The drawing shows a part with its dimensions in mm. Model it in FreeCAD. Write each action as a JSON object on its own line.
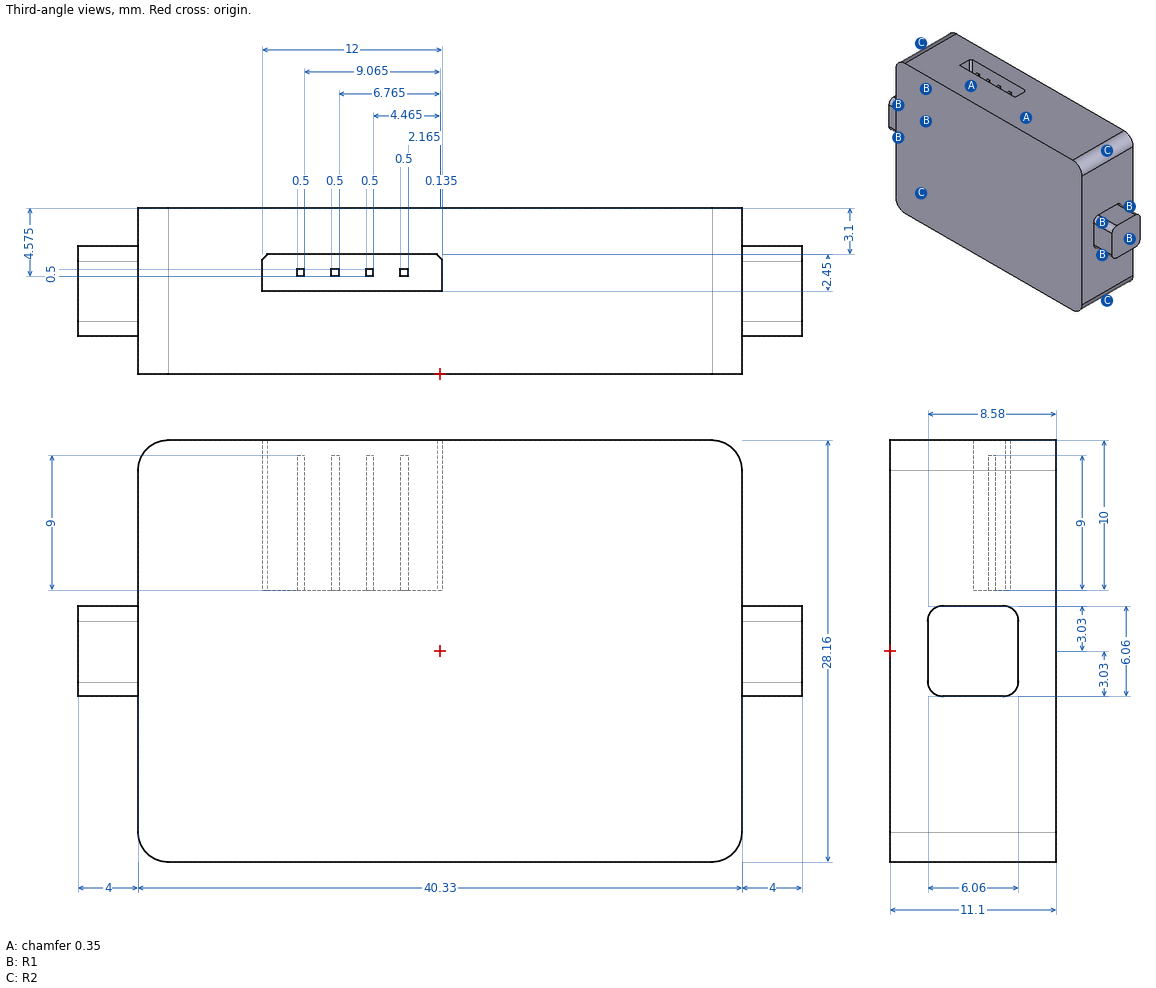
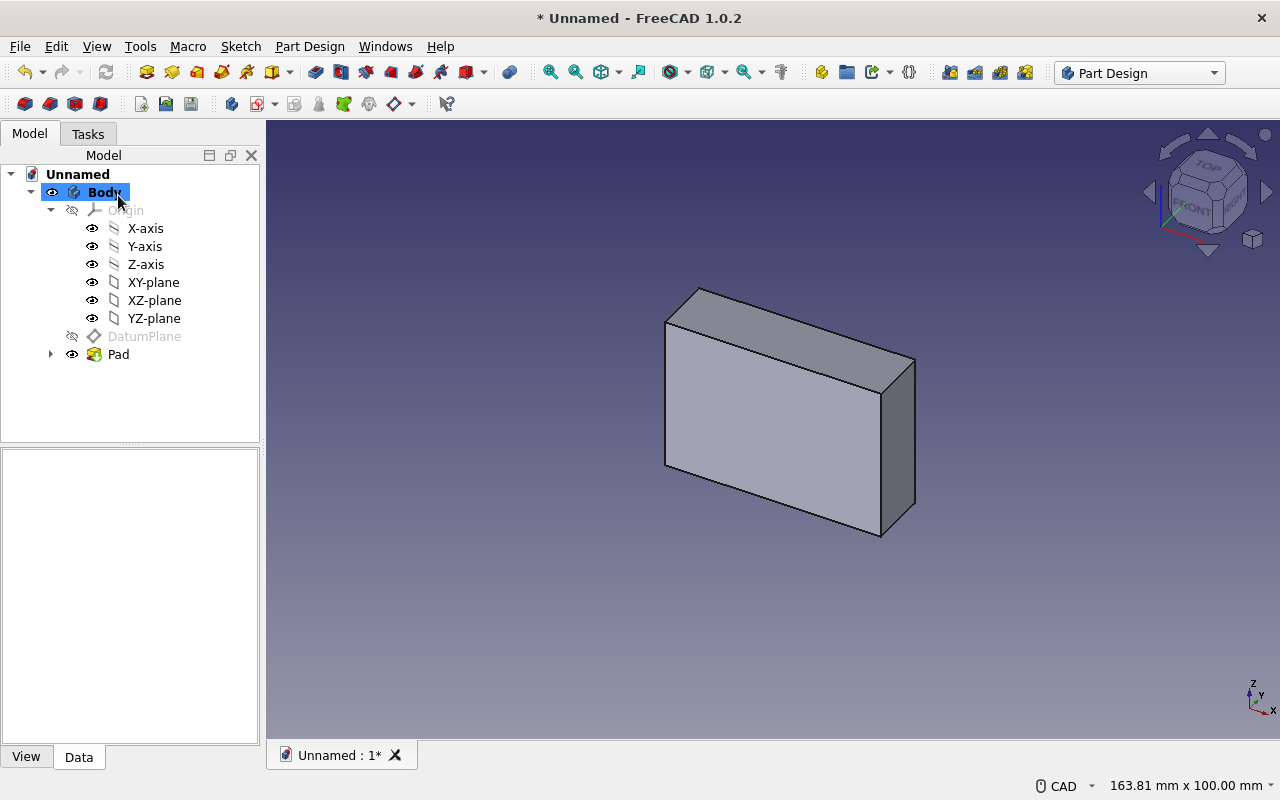
{"action": "key", "text": "v f"}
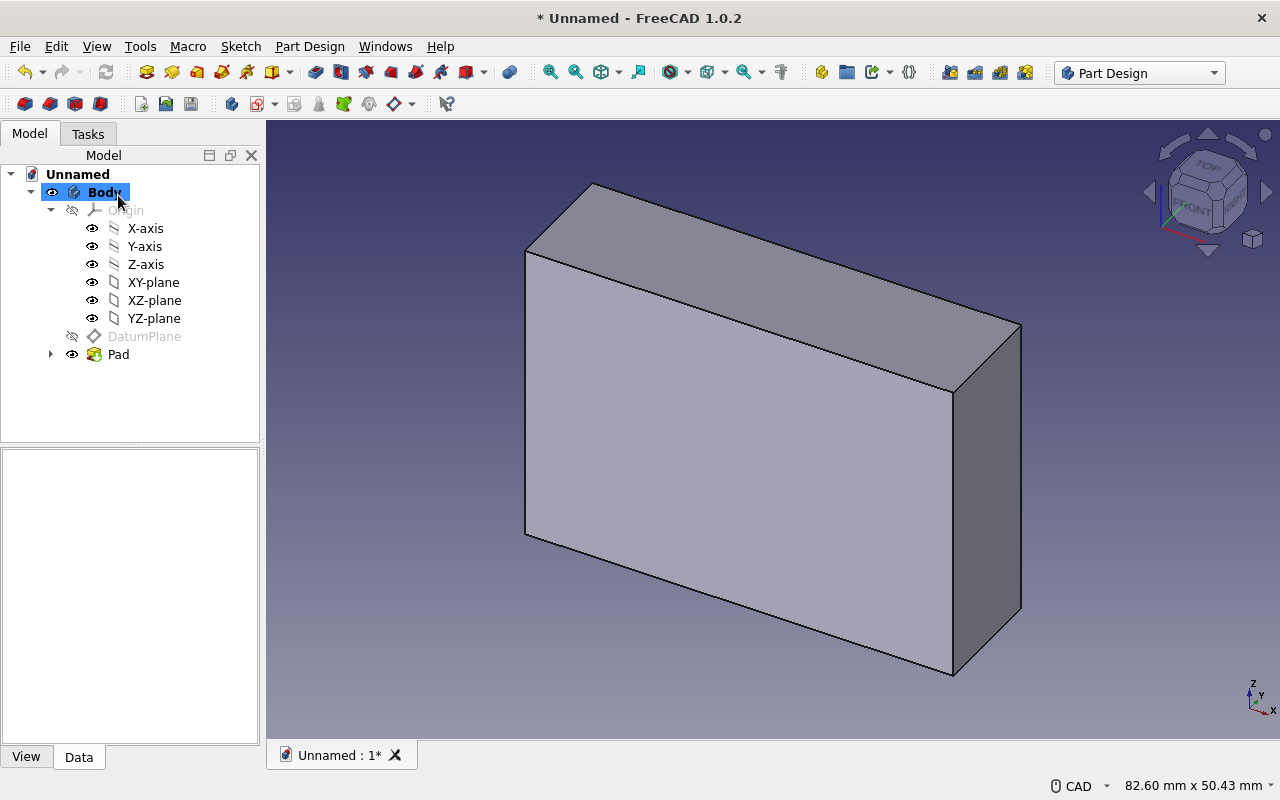
{"action": "left_click", "coordinate": [895, 327]}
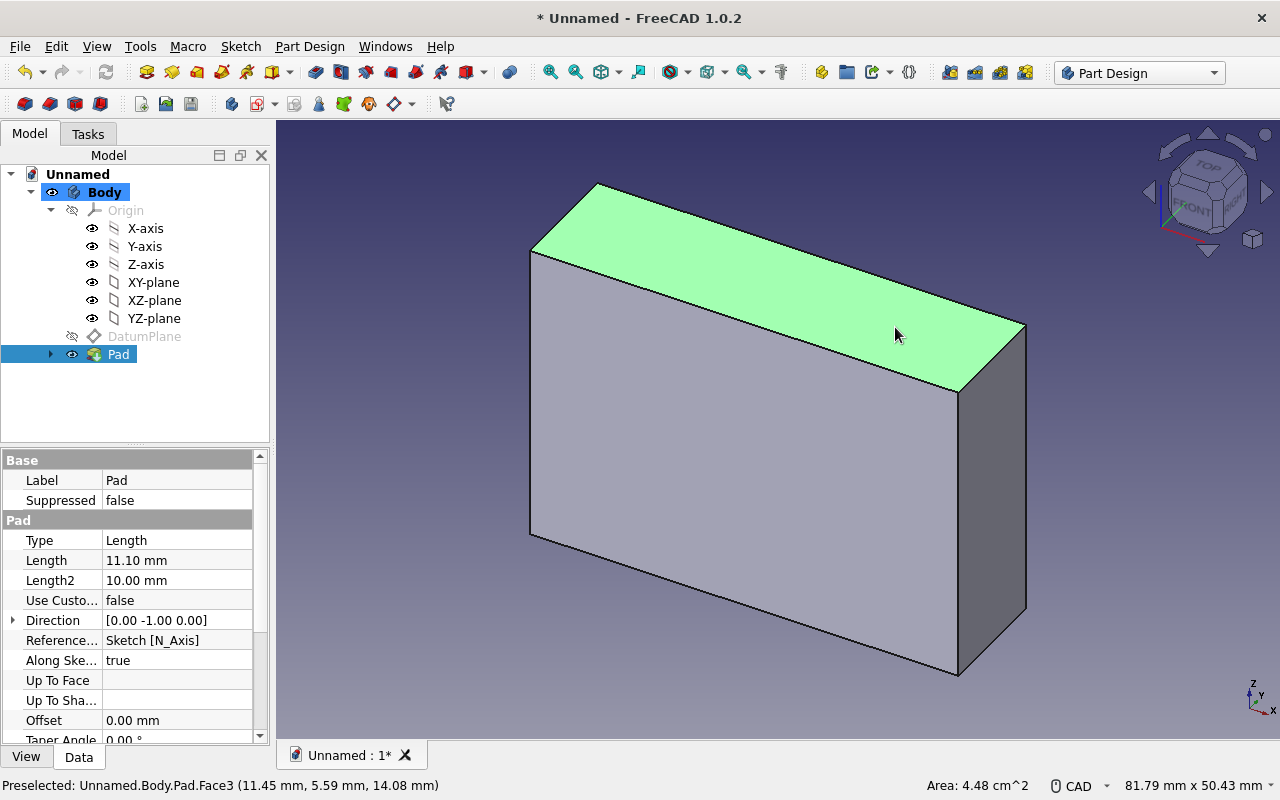
{"action": "left_click", "coordinate": [256, 104]}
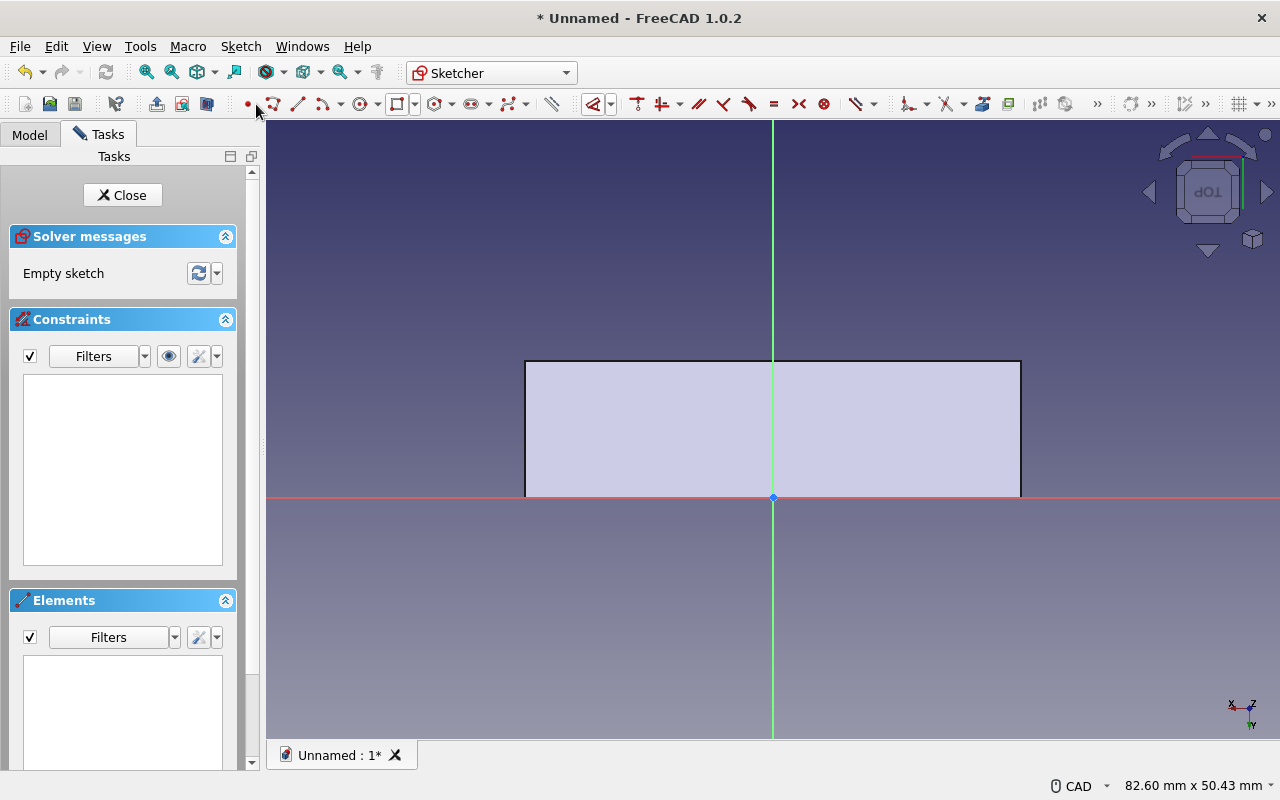
{"action": "scroll", "coordinate": [891, 475], "scroll_direction": "up", "scroll_amount": 7}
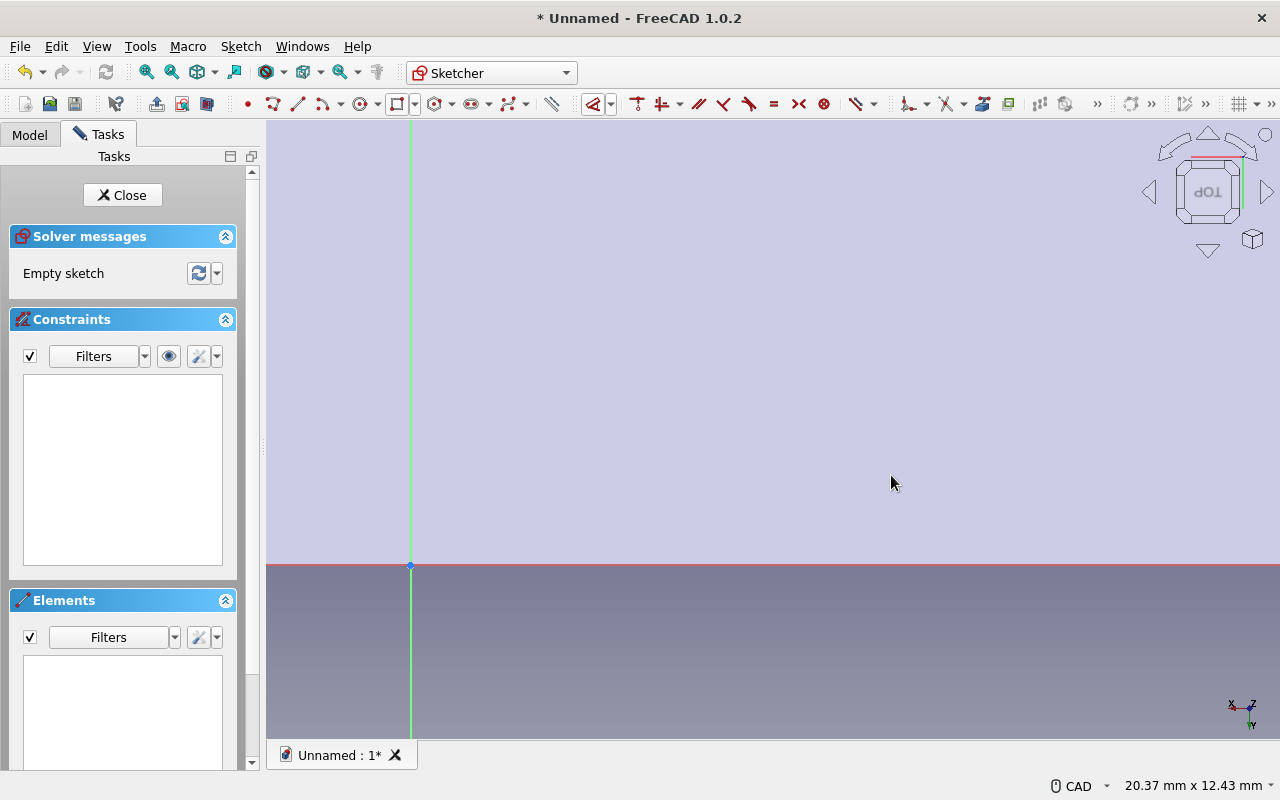
{"action": "left_click", "coordinate": [396, 104]}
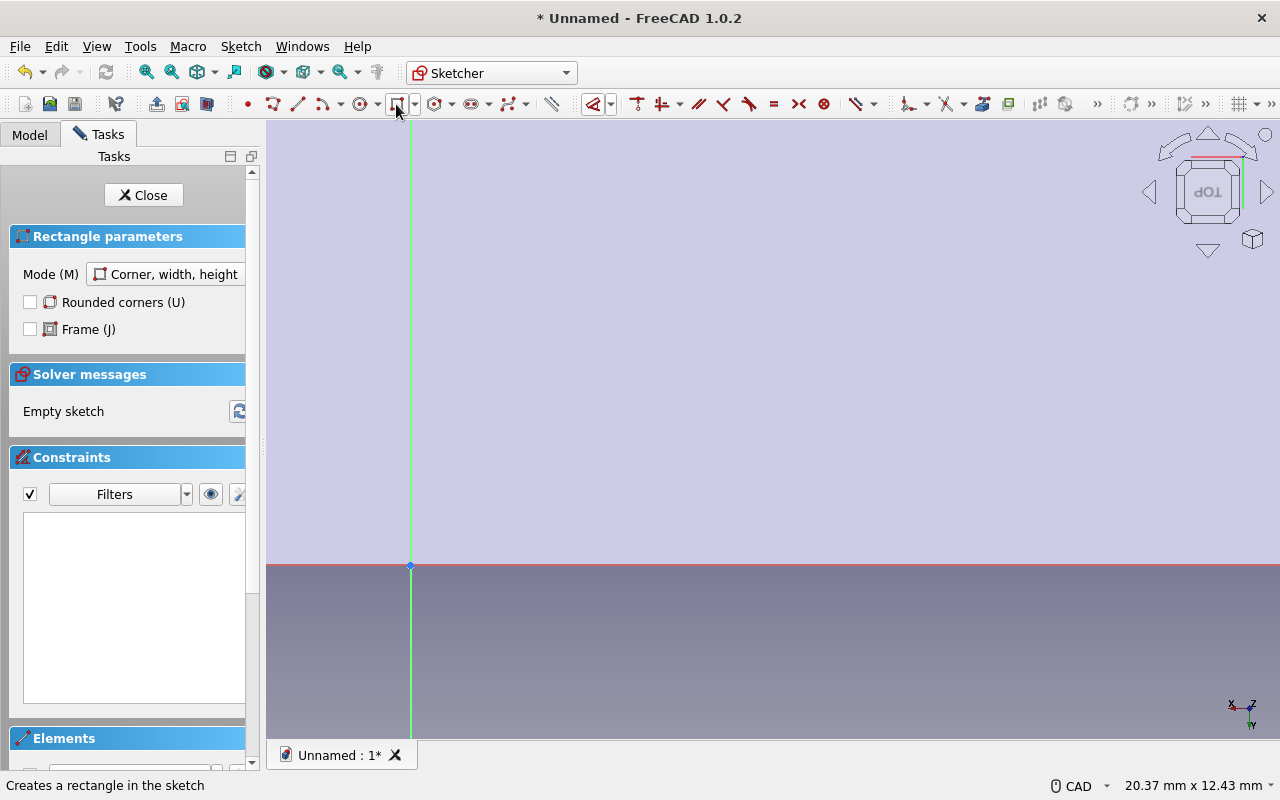
{"action": "scroll", "coordinate": [404, 289], "scroll_direction": "up", "scroll_amount": 5}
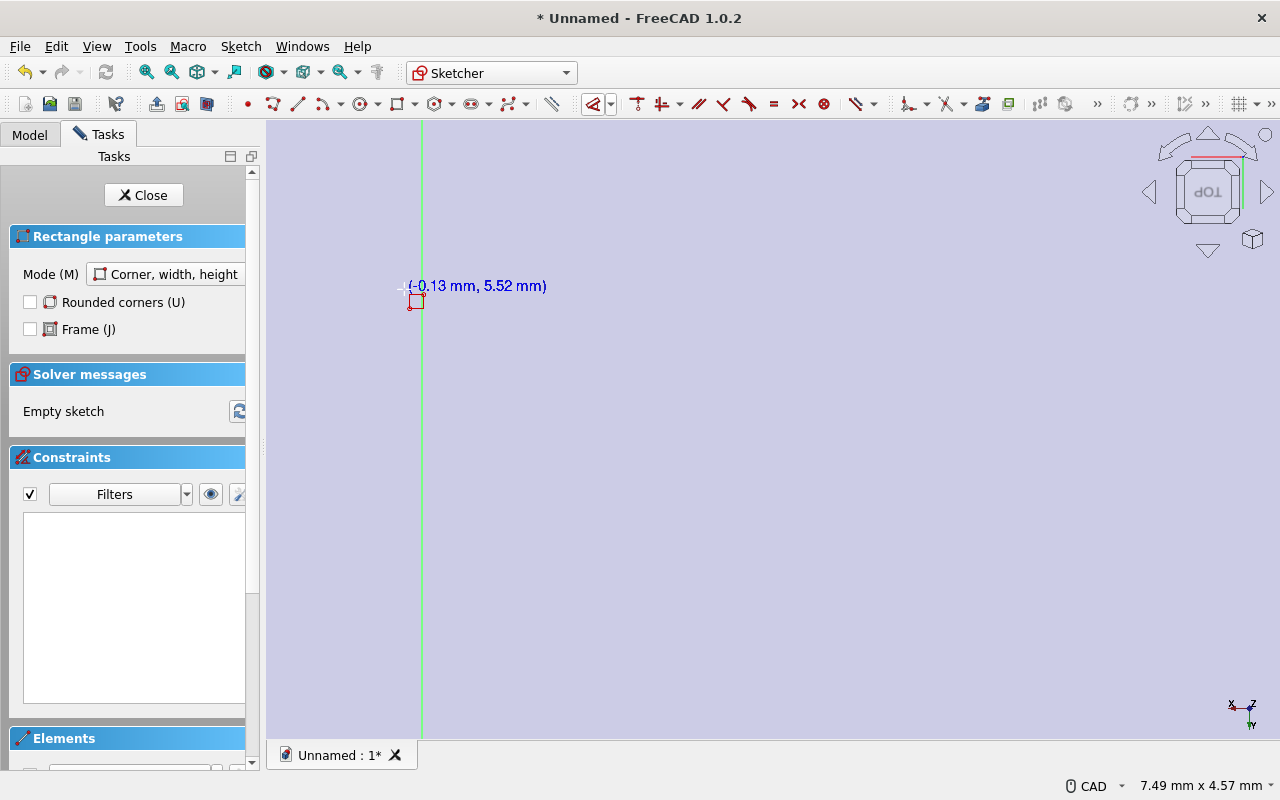
{"action": "left_click", "coordinate": [403, 288]}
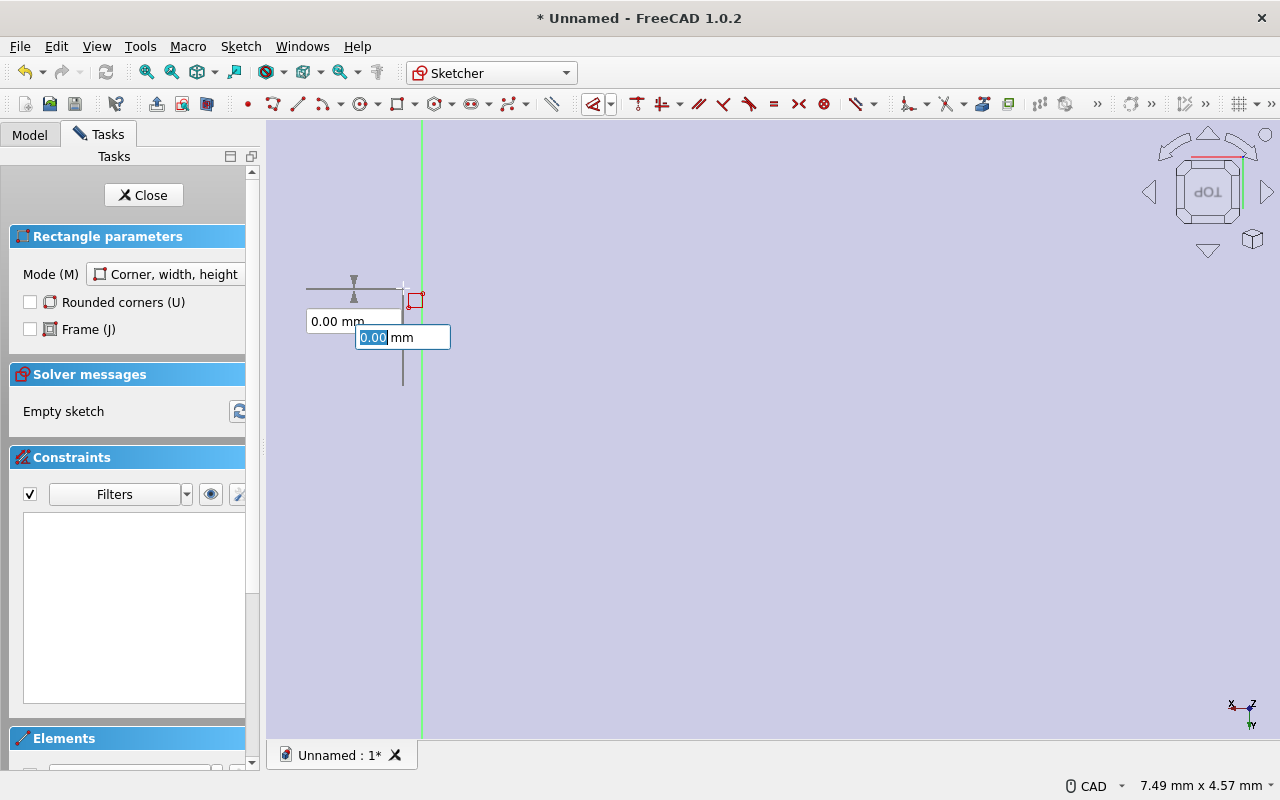
{"action": "scroll", "coordinate": [407, 293], "scroll_direction": "down", "scroll_amount": 5}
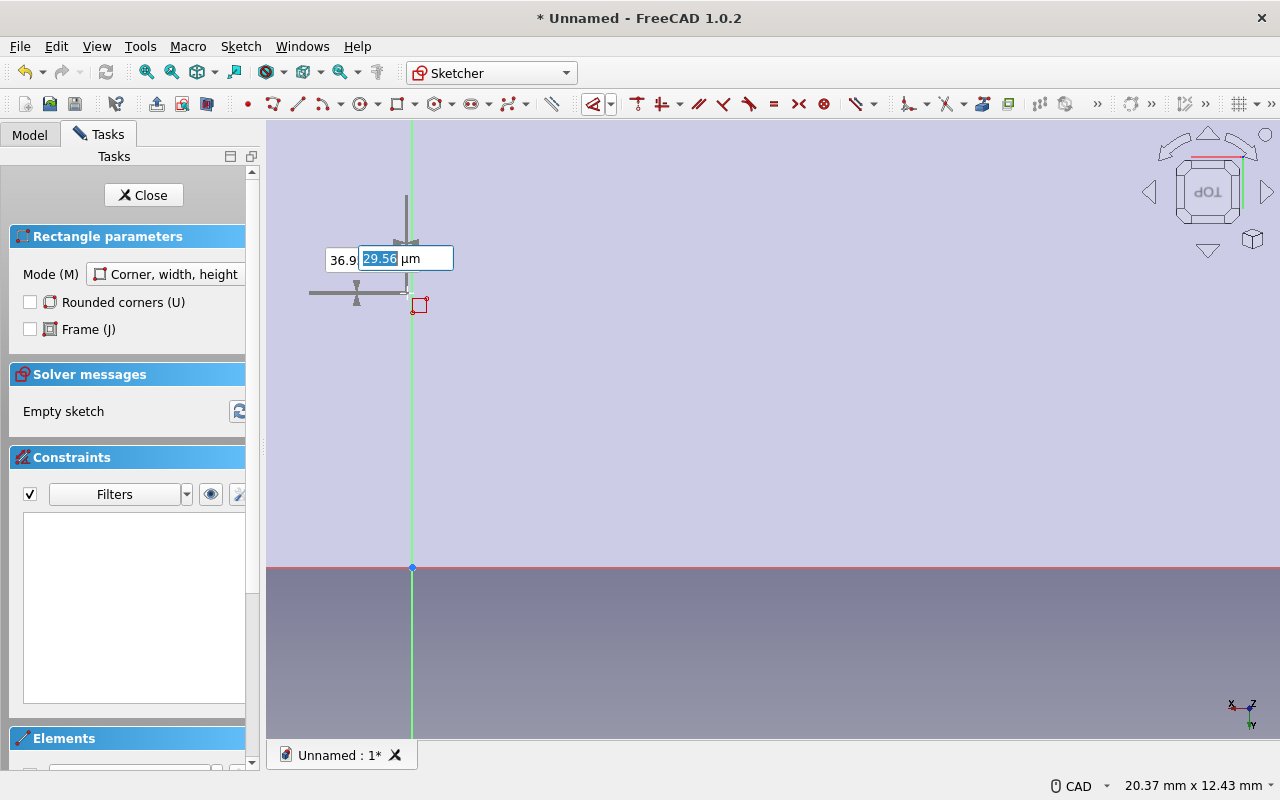
{"action": "left_click", "coordinate": [1003, 413]}
{"action": "key", "text": "Escape"}